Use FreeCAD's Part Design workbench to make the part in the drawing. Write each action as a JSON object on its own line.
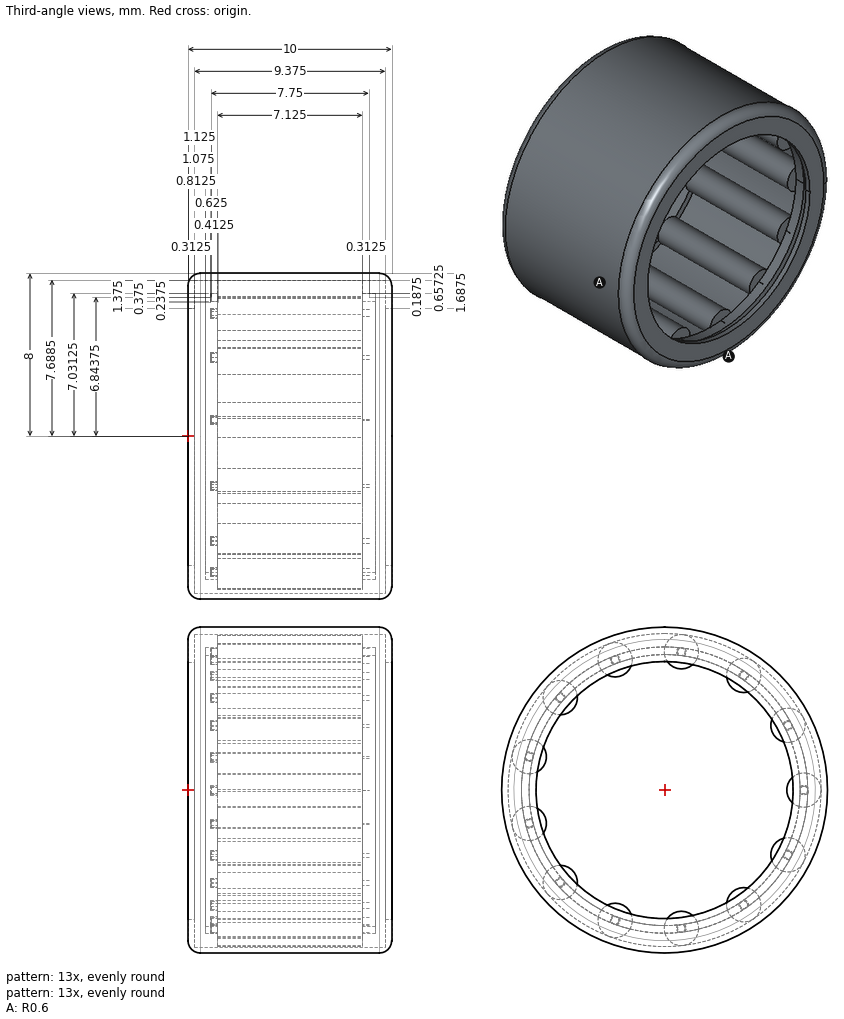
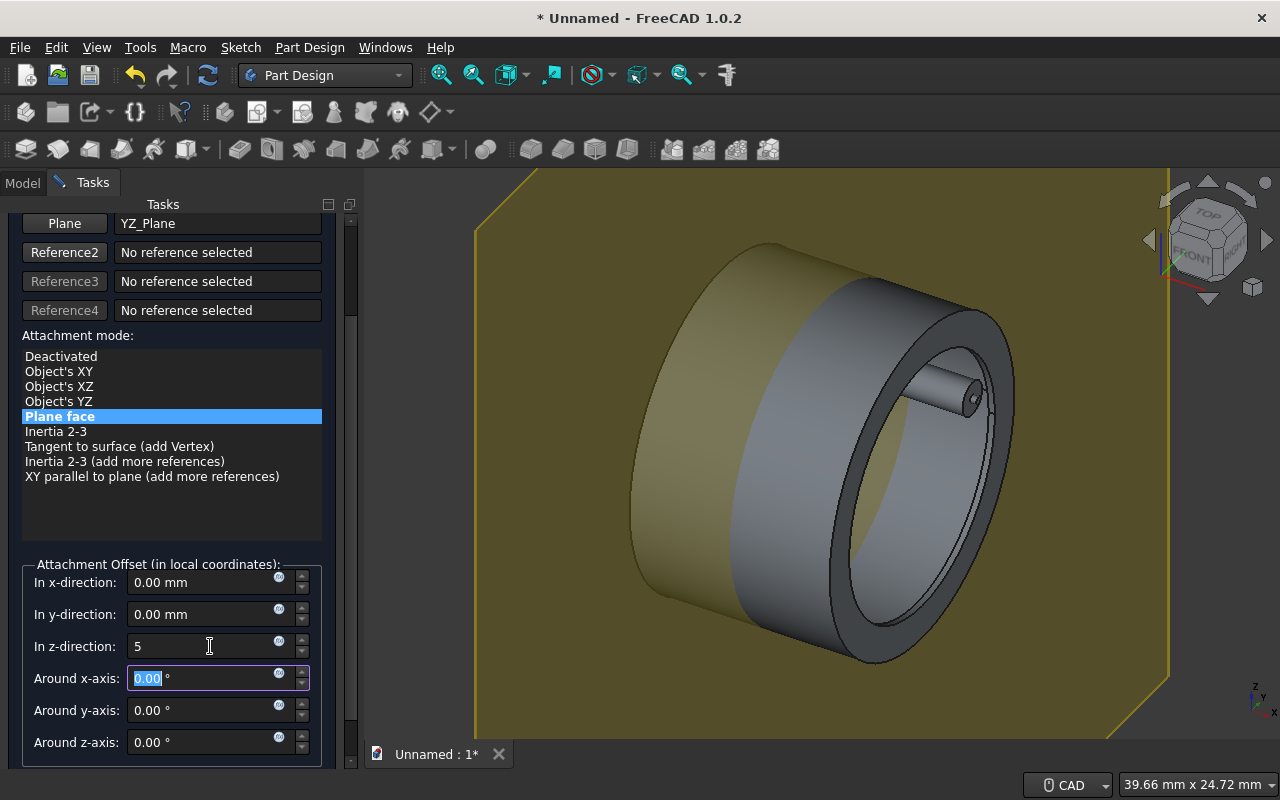
{"action": "scroll", "coordinate": [351, 491], "scroll_direction": "up", "scroll_amount": 3}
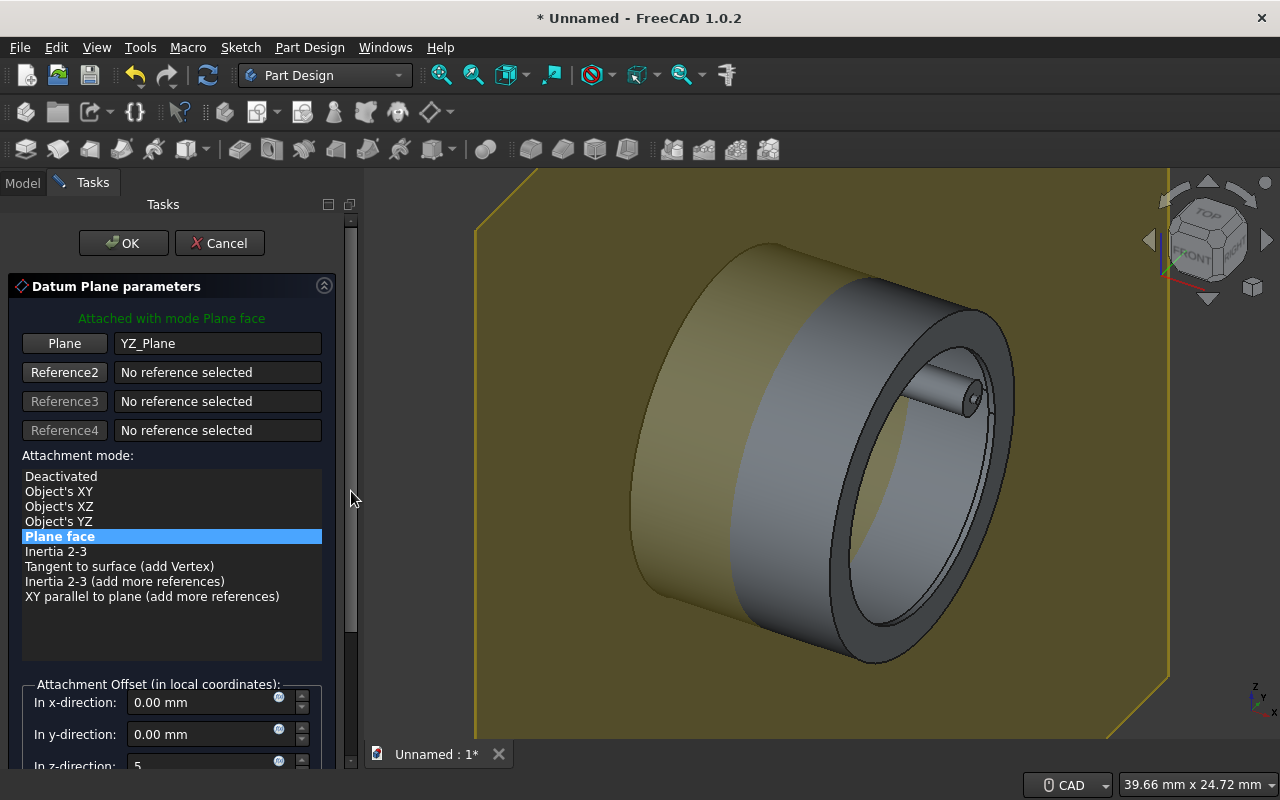
{"action": "left_click", "coordinate": [124, 243]}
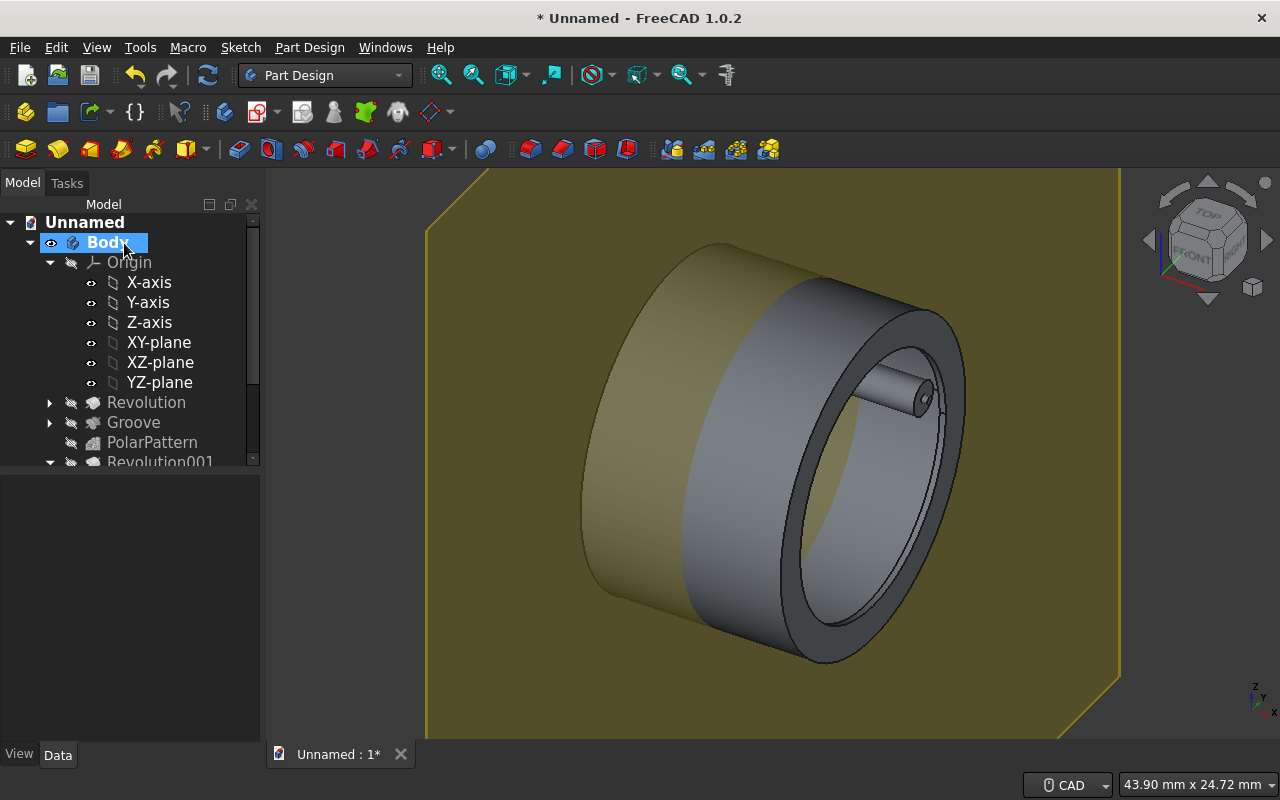
{"action": "left_click", "coordinate": [116, 403]}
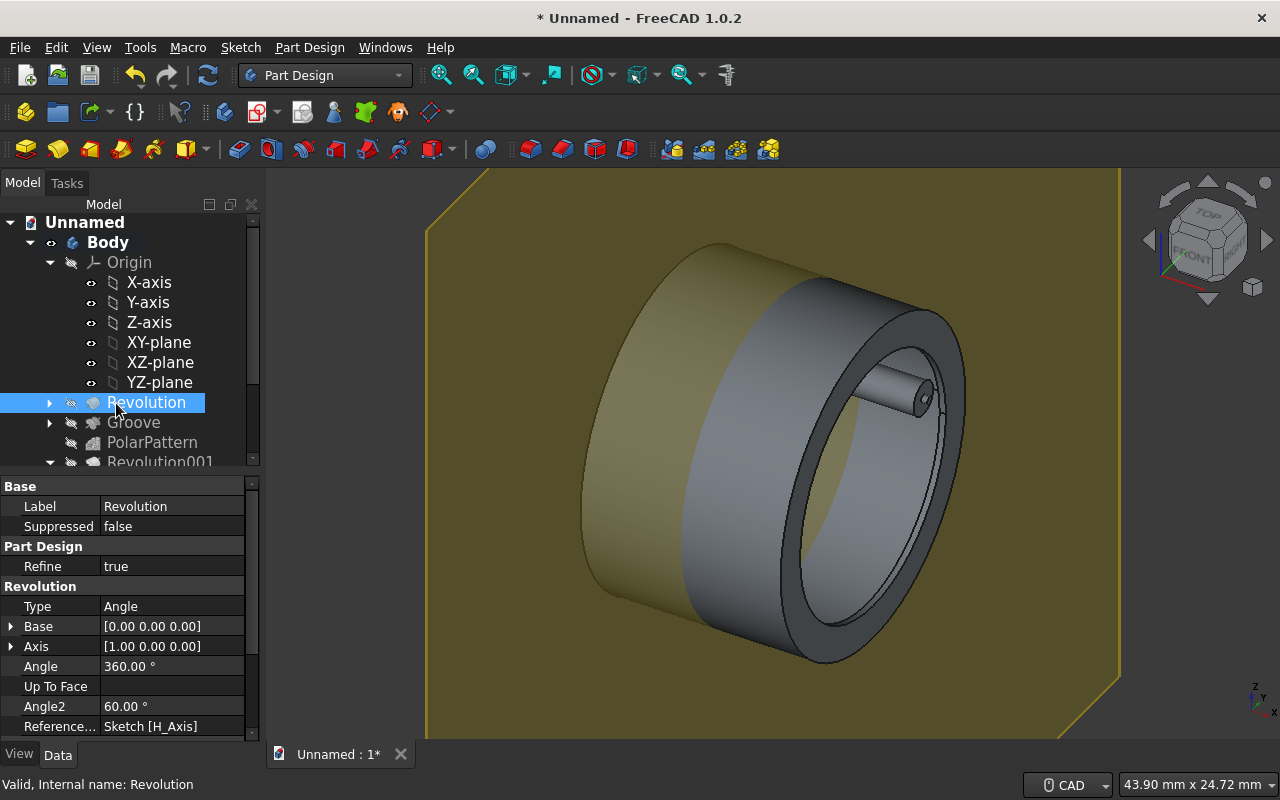
{"action": "left_click", "coordinate": [672, 150]}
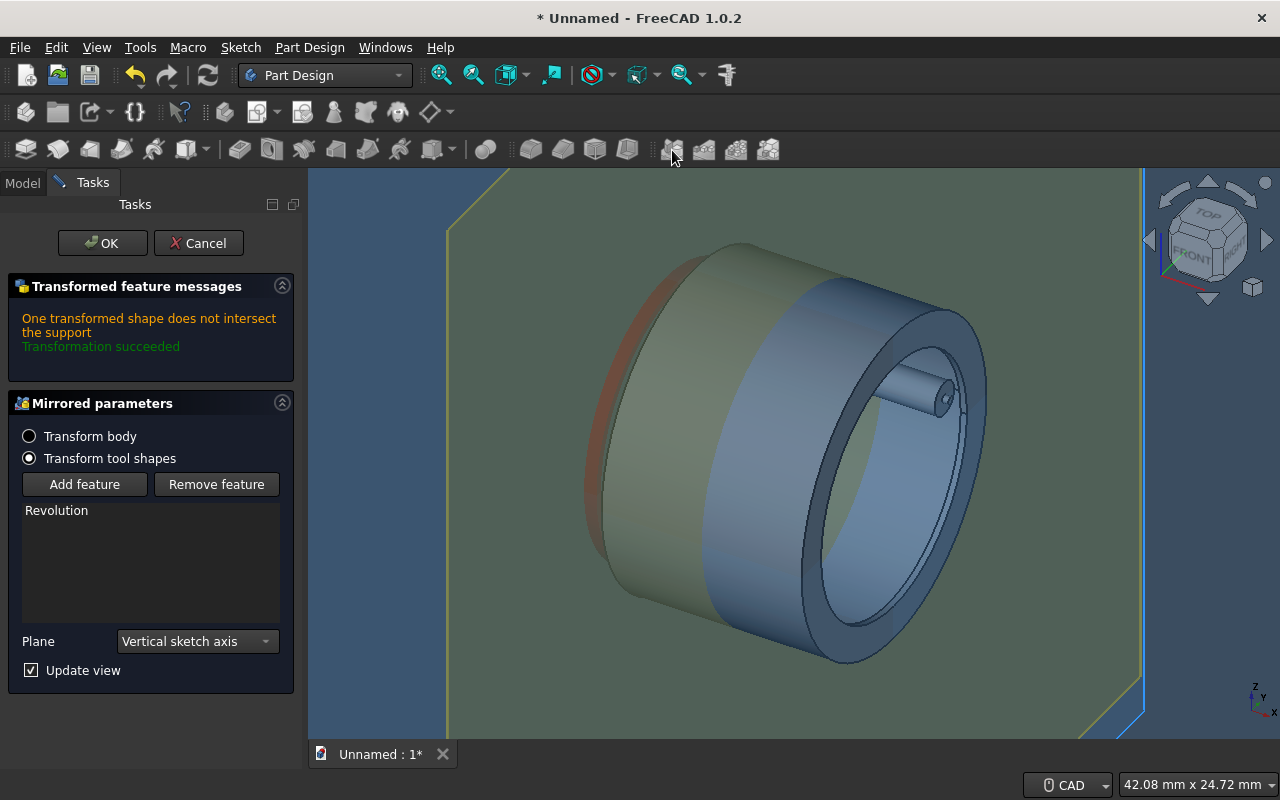
{"action": "left_click", "coordinate": [198, 642]}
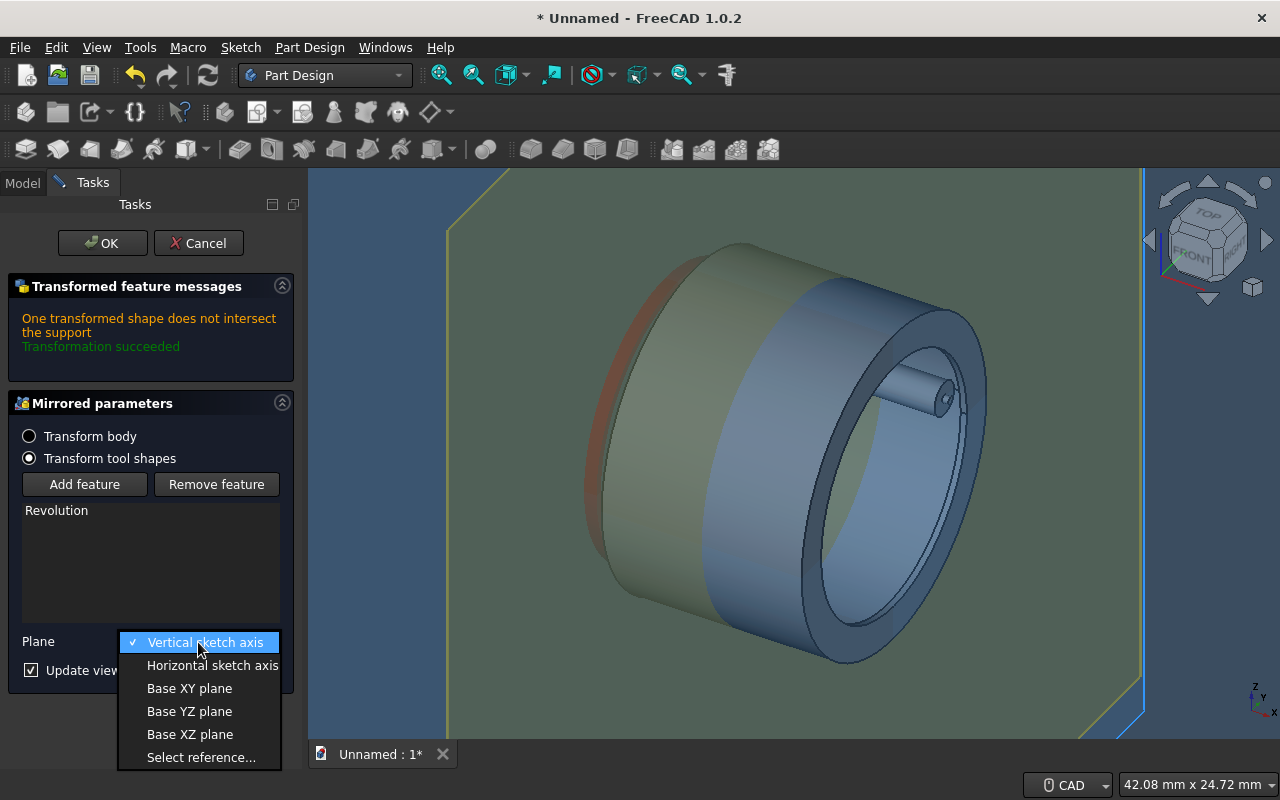
{"action": "left_click", "coordinate": [198, 758]}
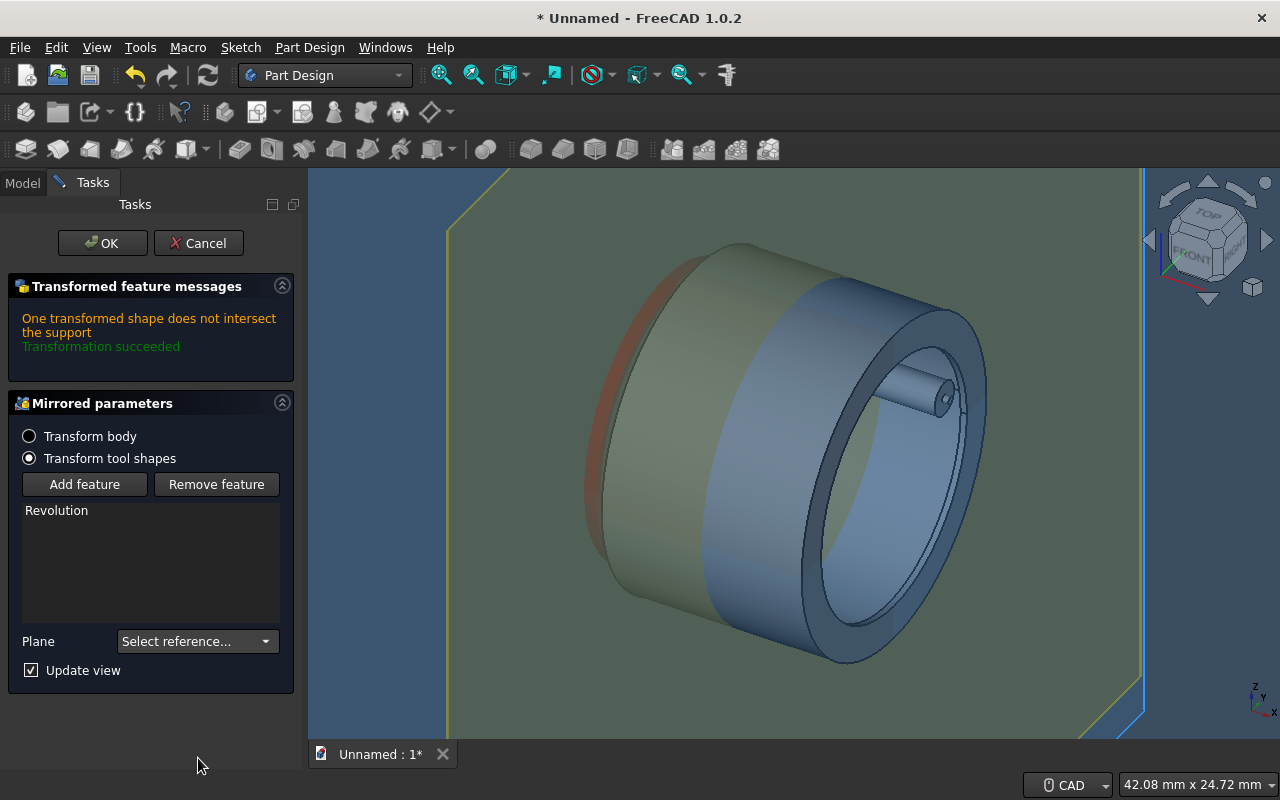
{"action": "left_click", "coordinate": [23, 182]}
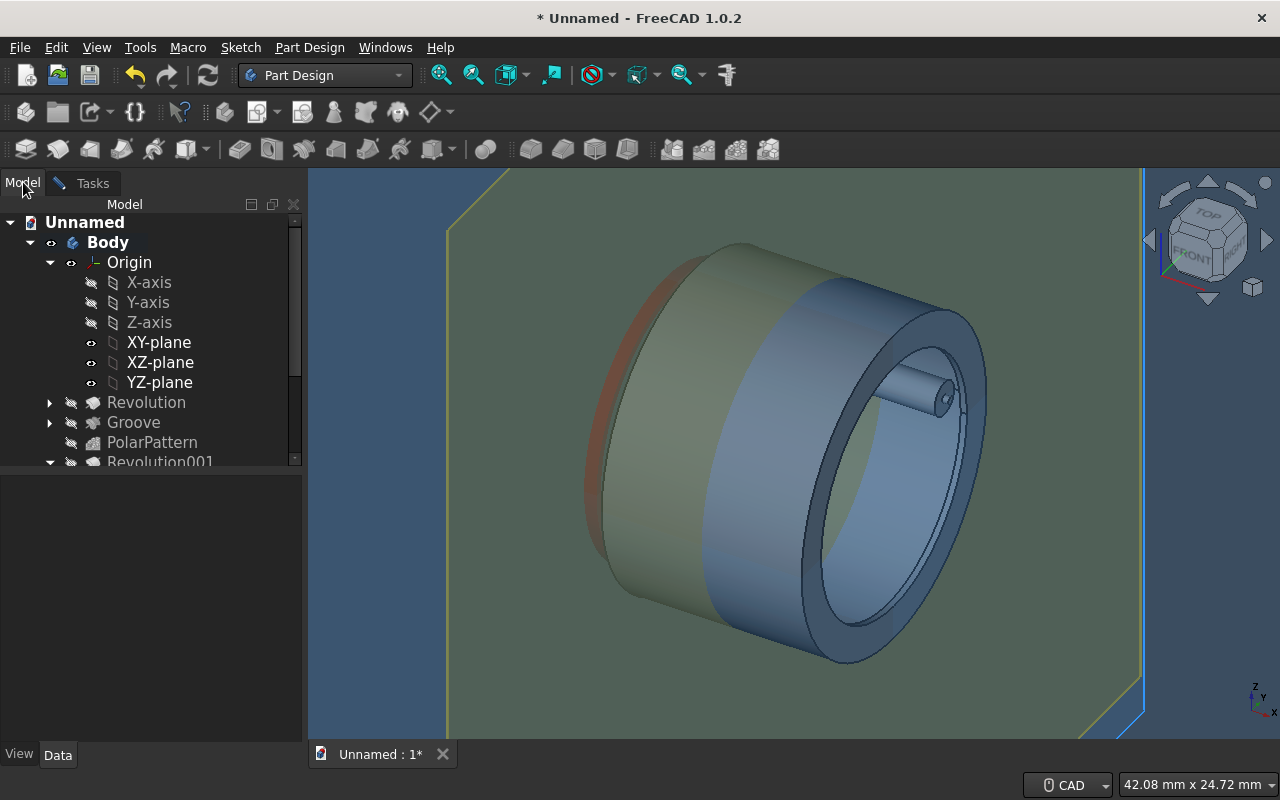
{"action": "scroll", "coordinate": [100, 338], "scroll_direction": "down", "scroll_amount": 3}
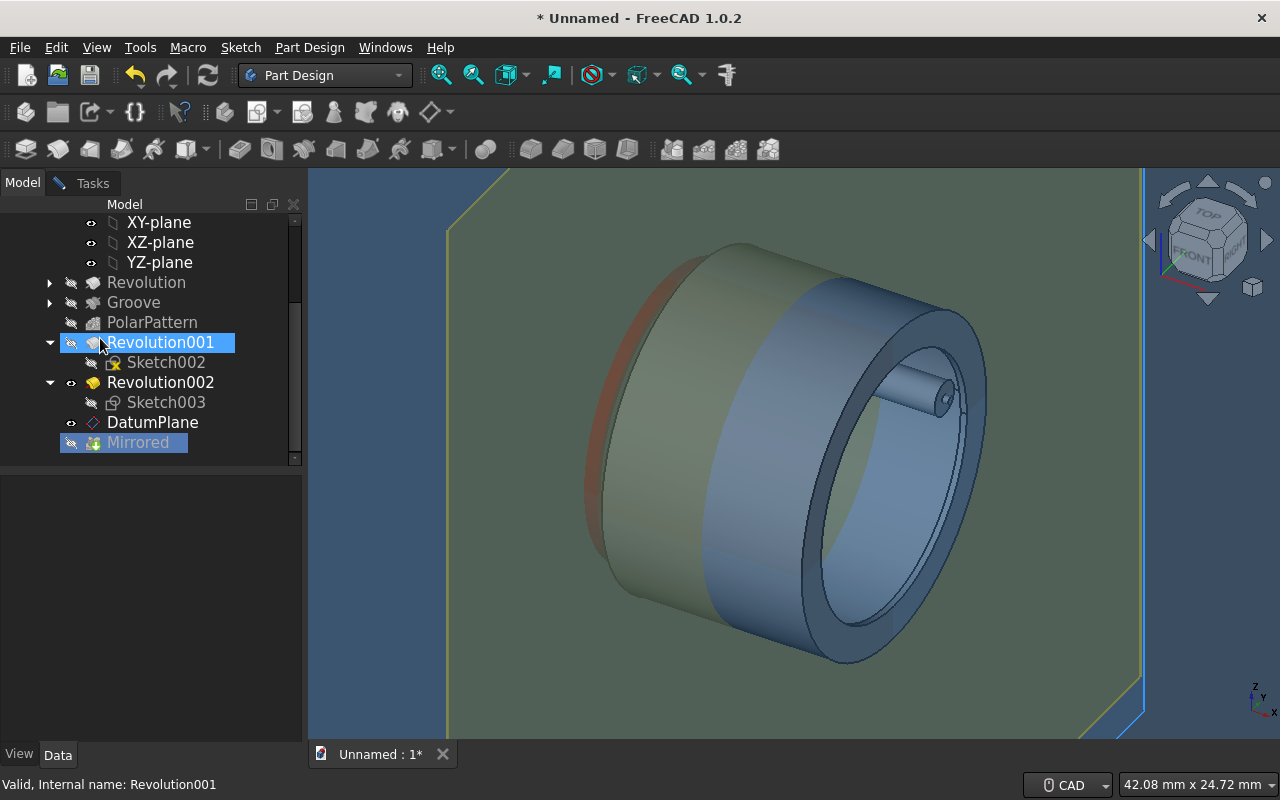
{"action": "left_click", "coordinate": [116, 423]}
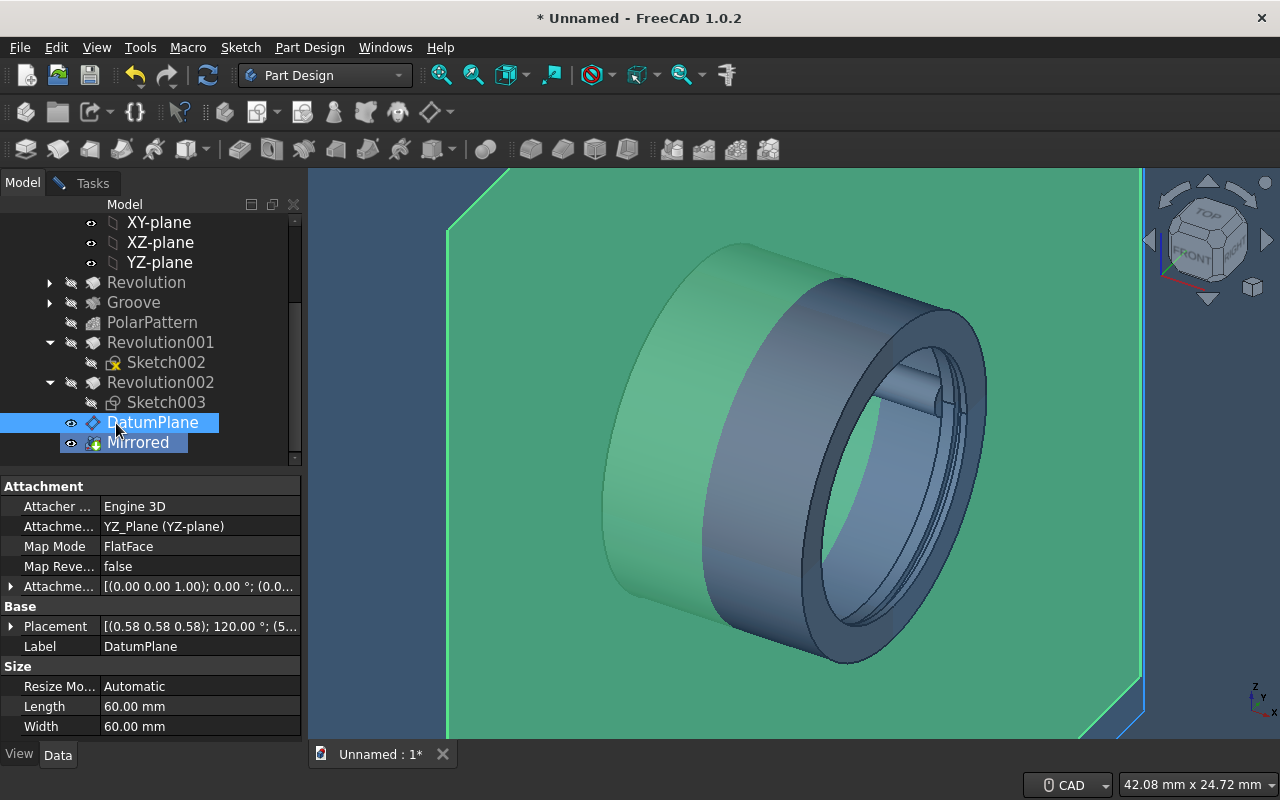
{"action": "left_click", "coordinate": [84, 182]}